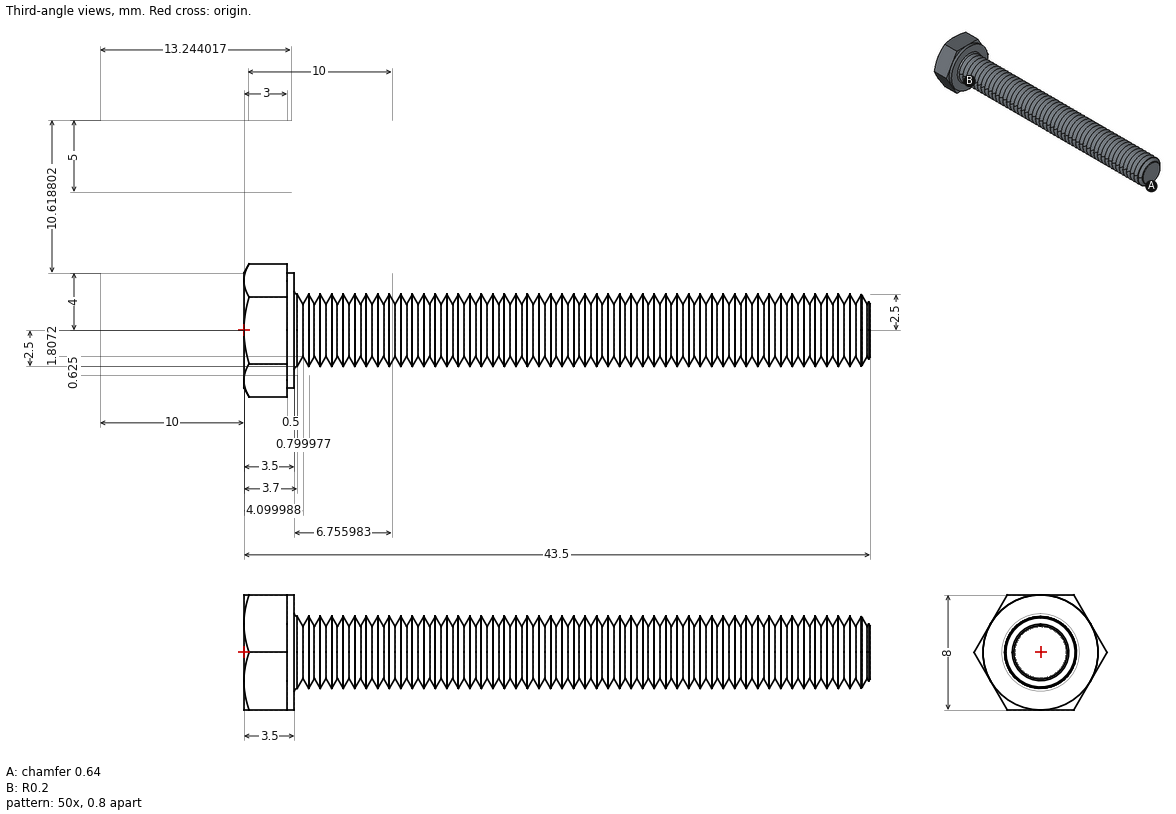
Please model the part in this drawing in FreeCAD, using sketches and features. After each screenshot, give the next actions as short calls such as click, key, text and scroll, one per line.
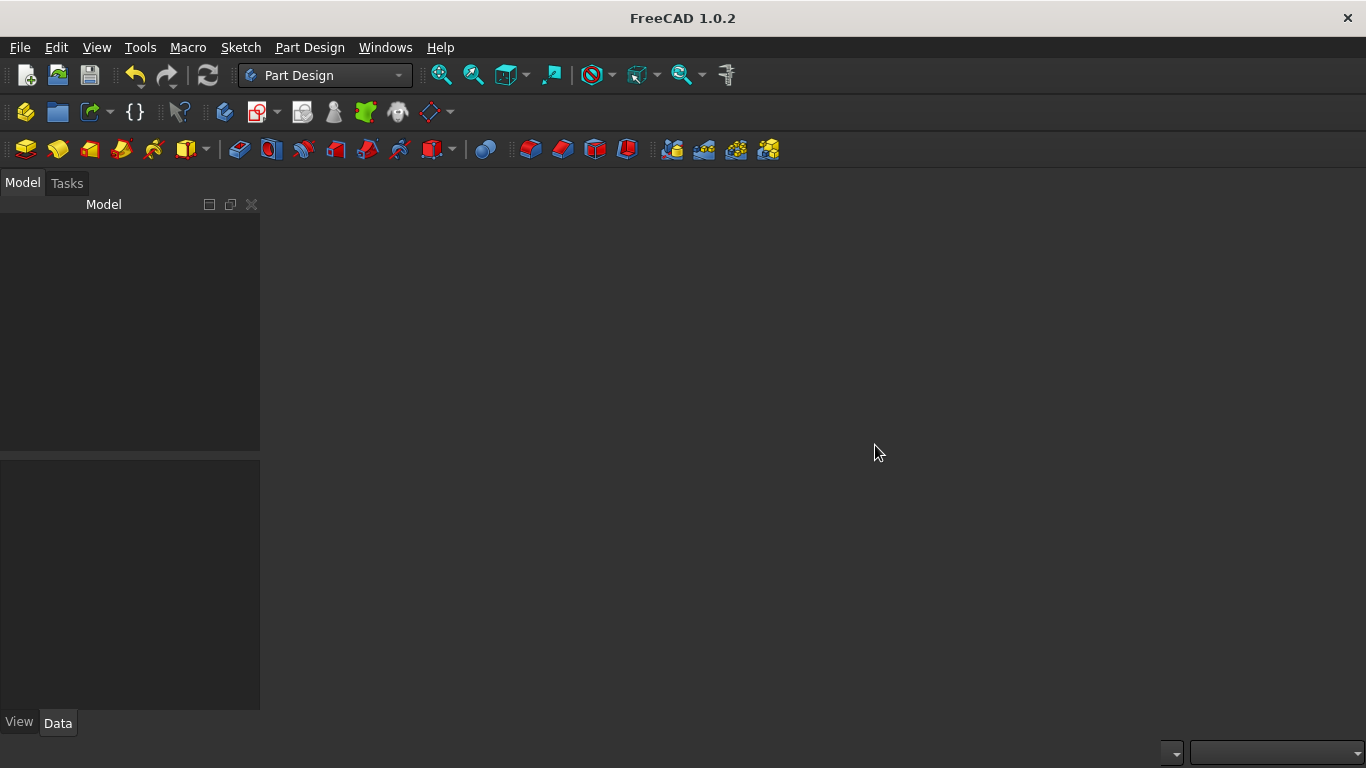
click(26, 76)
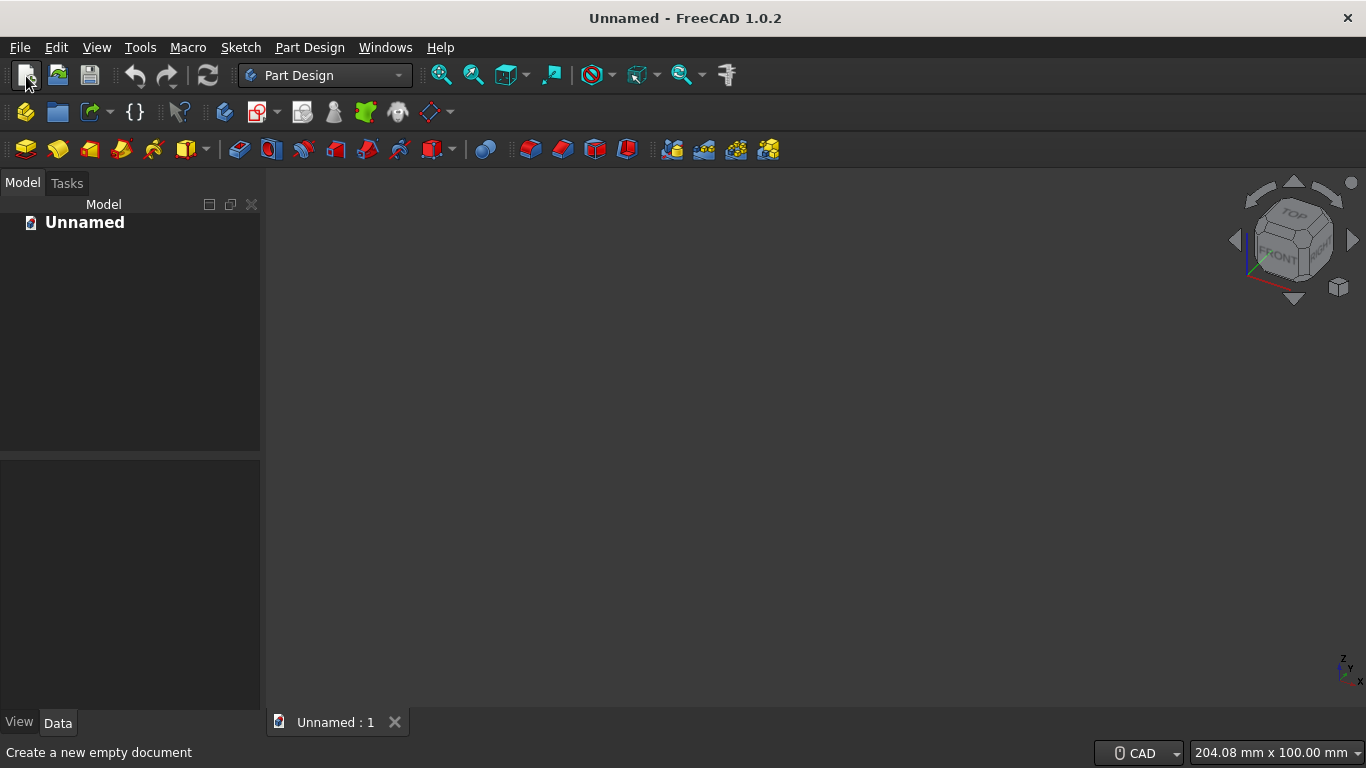
click(258, 112)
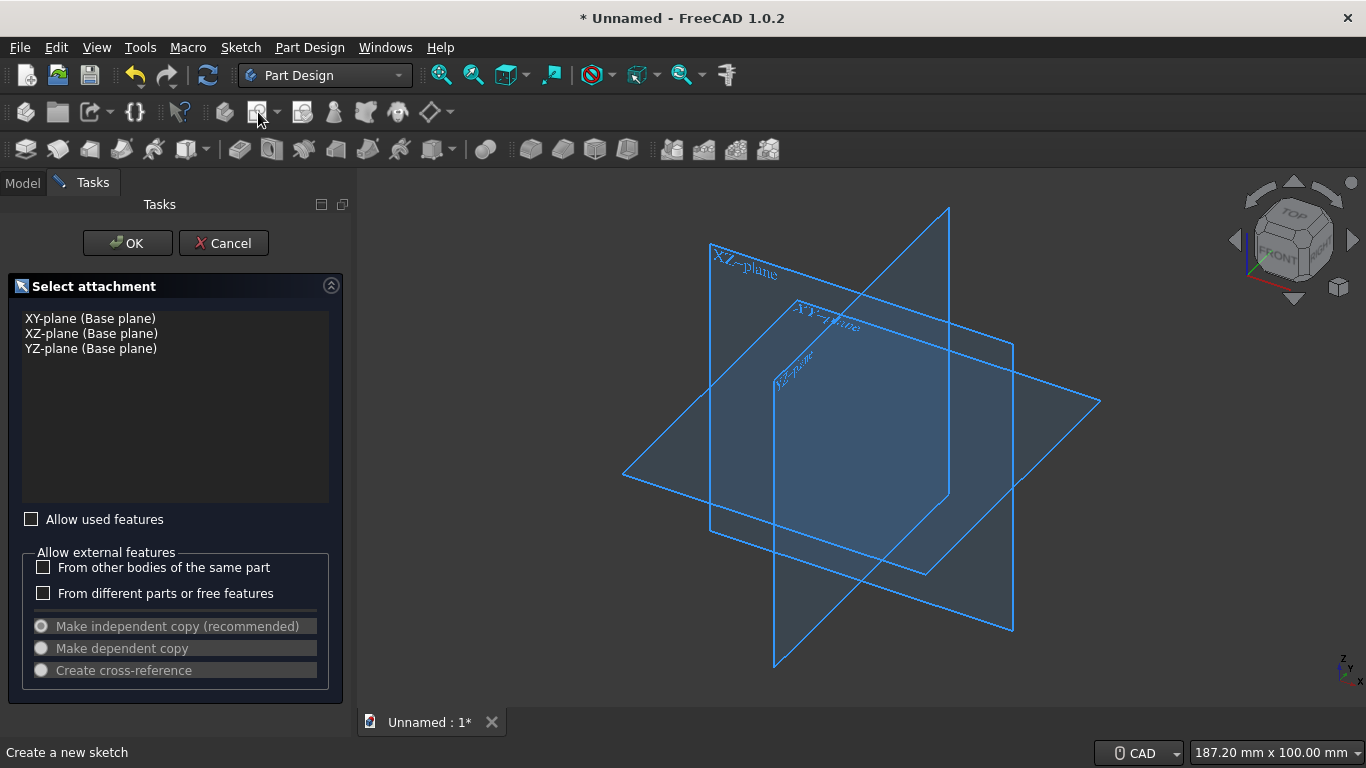
click(82, 348)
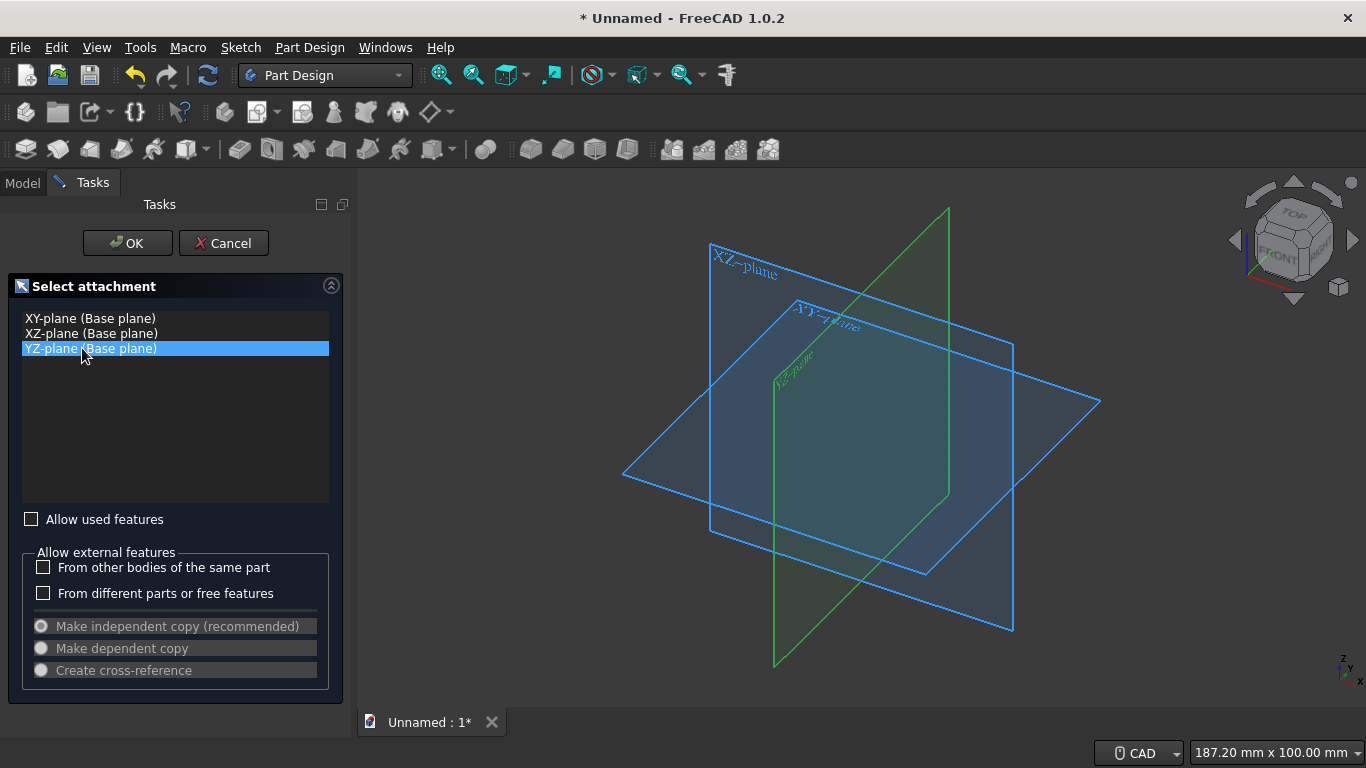
click(128, 243)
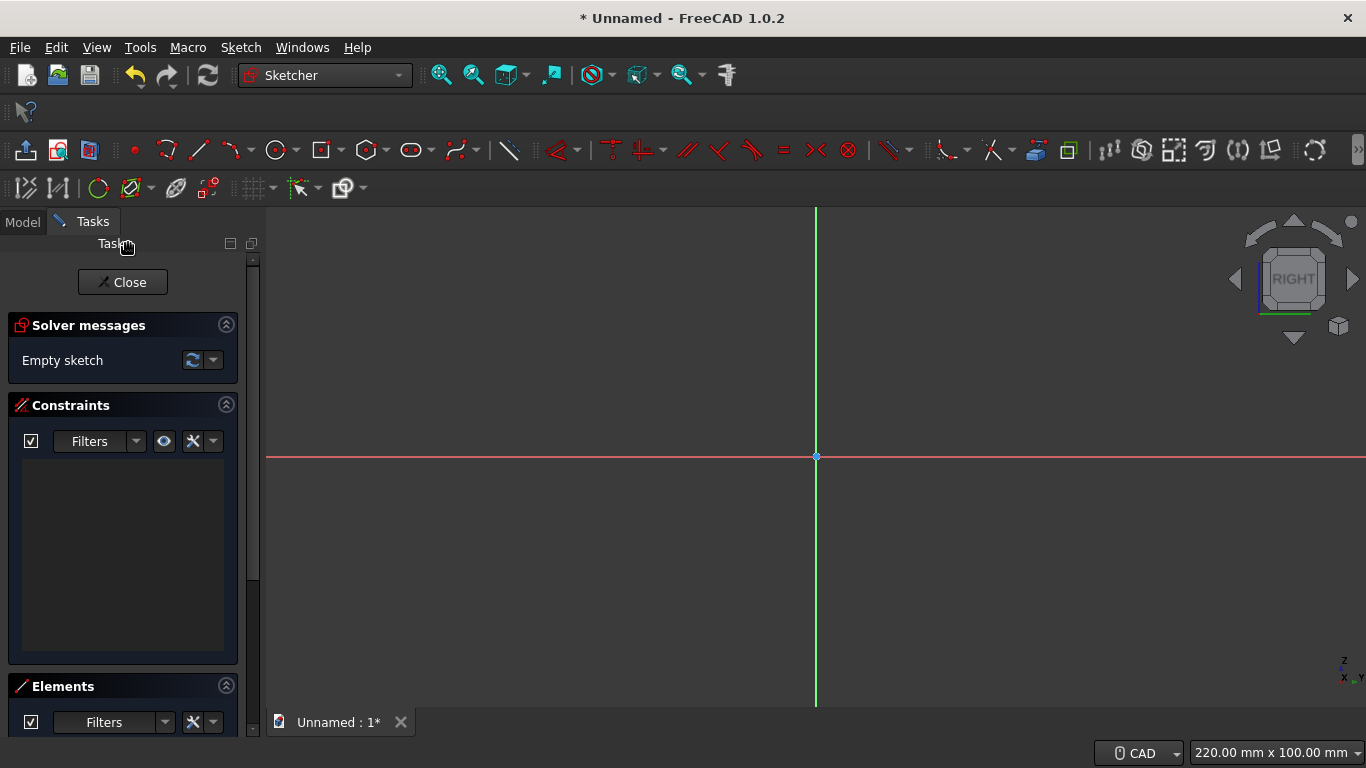
scroll(827, 457, up, 10)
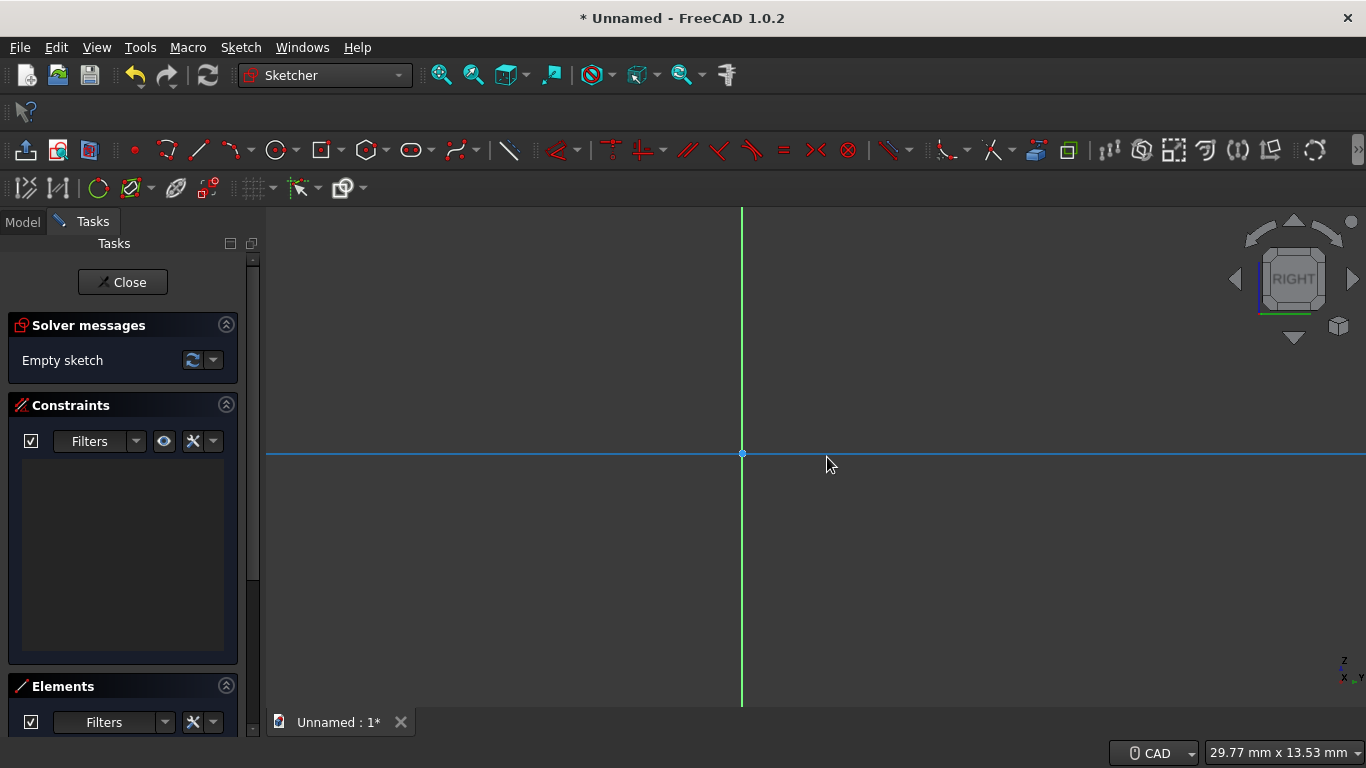
click(366, 150)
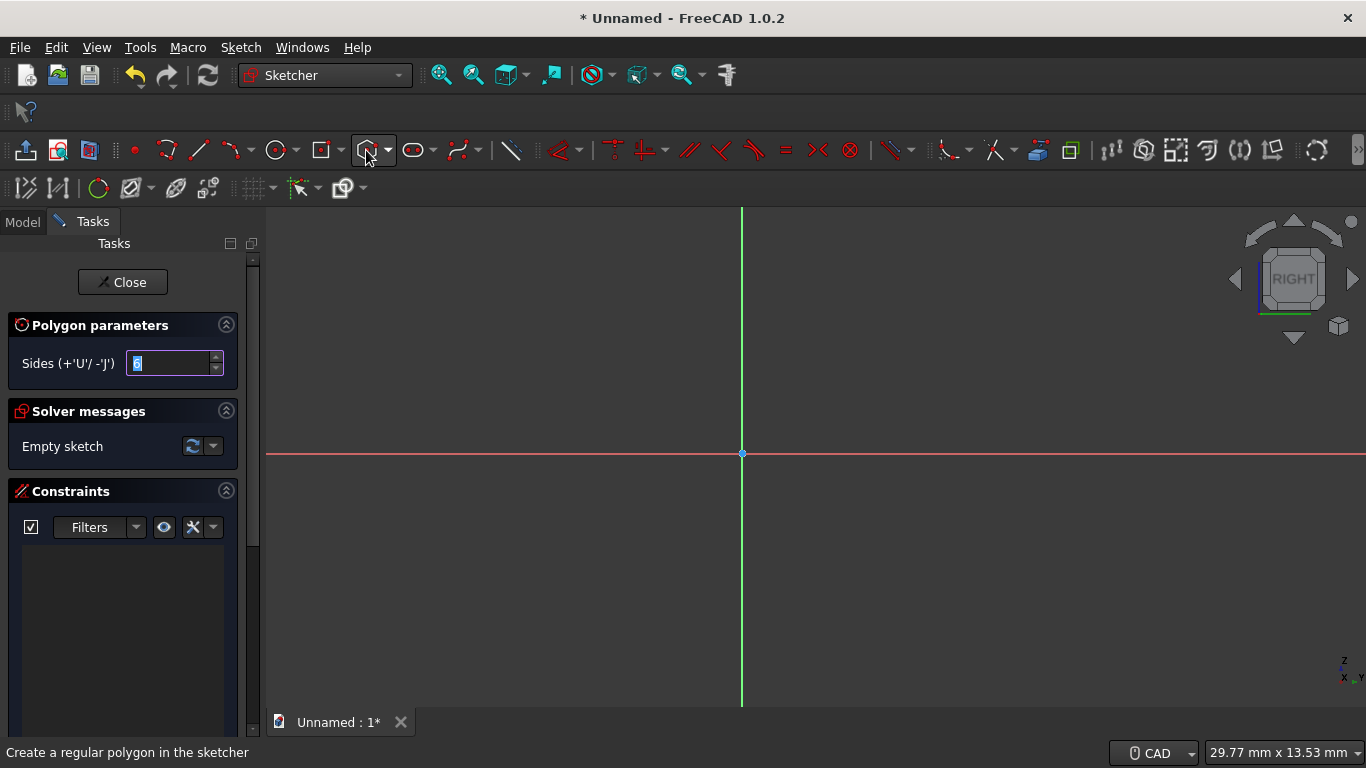
click(742, 454)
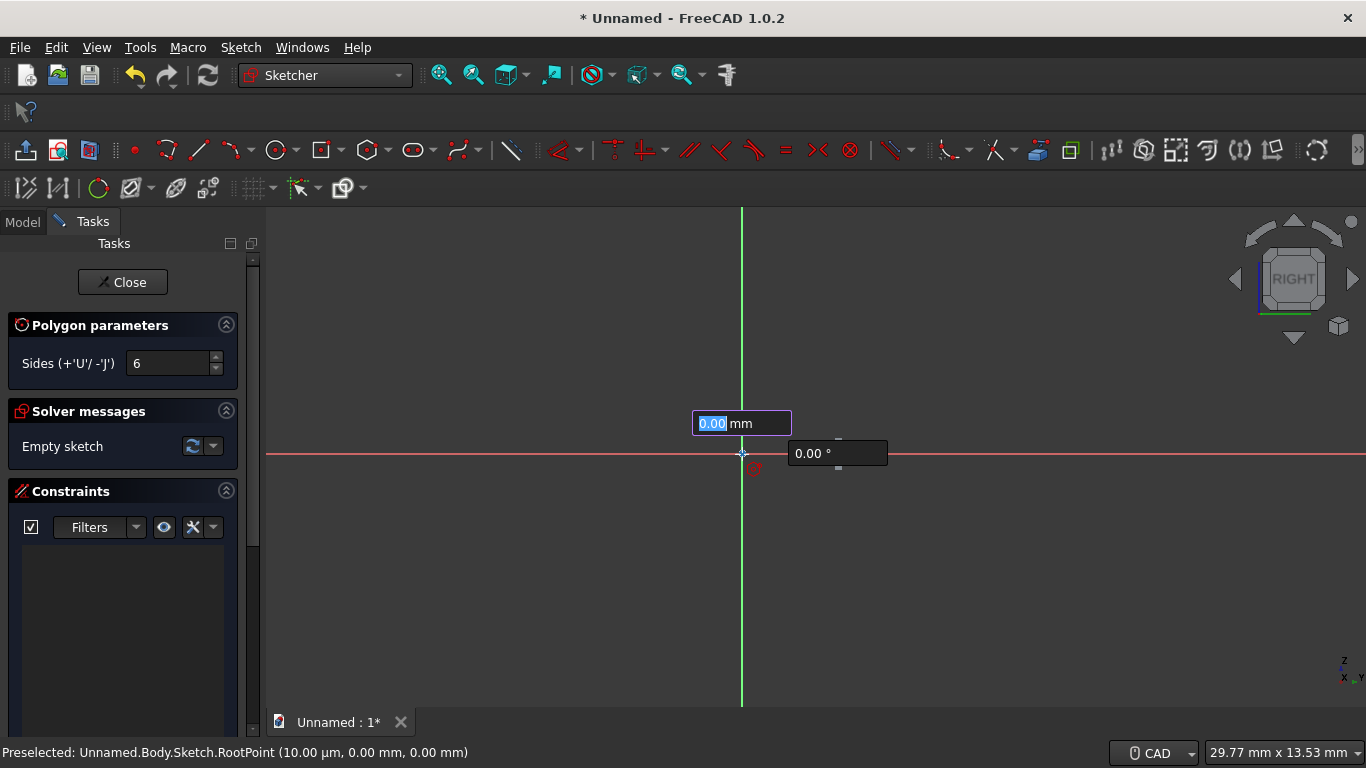
click(913, 454)
right_click(913, 454)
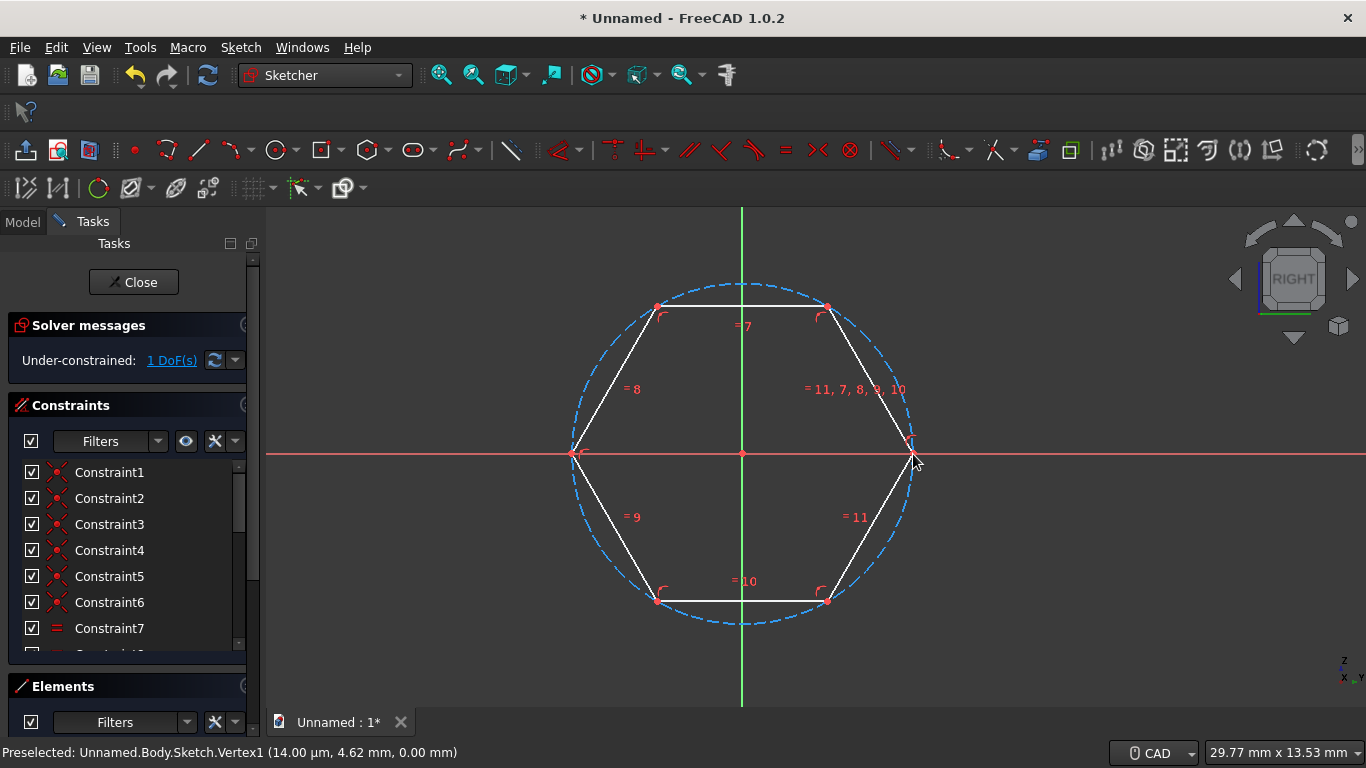
click(558, 150)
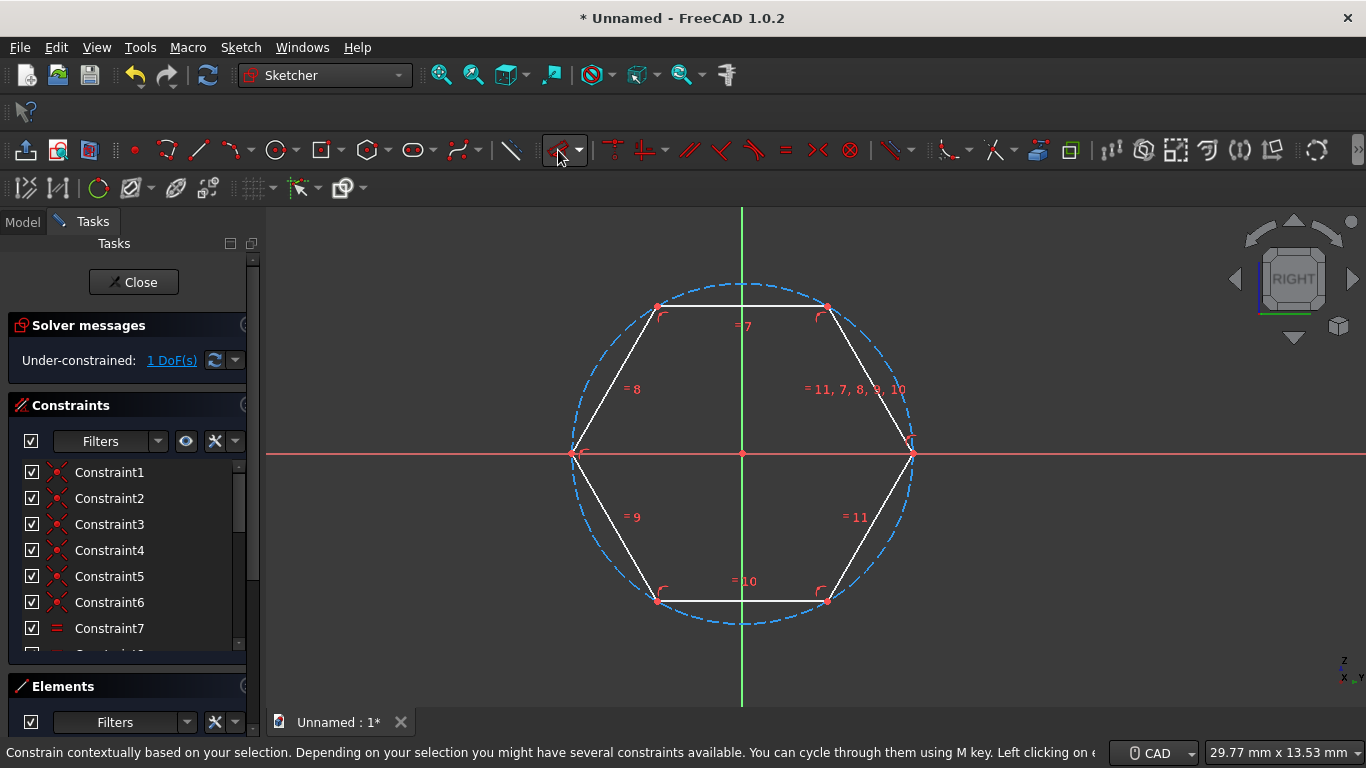
click(657, 601)